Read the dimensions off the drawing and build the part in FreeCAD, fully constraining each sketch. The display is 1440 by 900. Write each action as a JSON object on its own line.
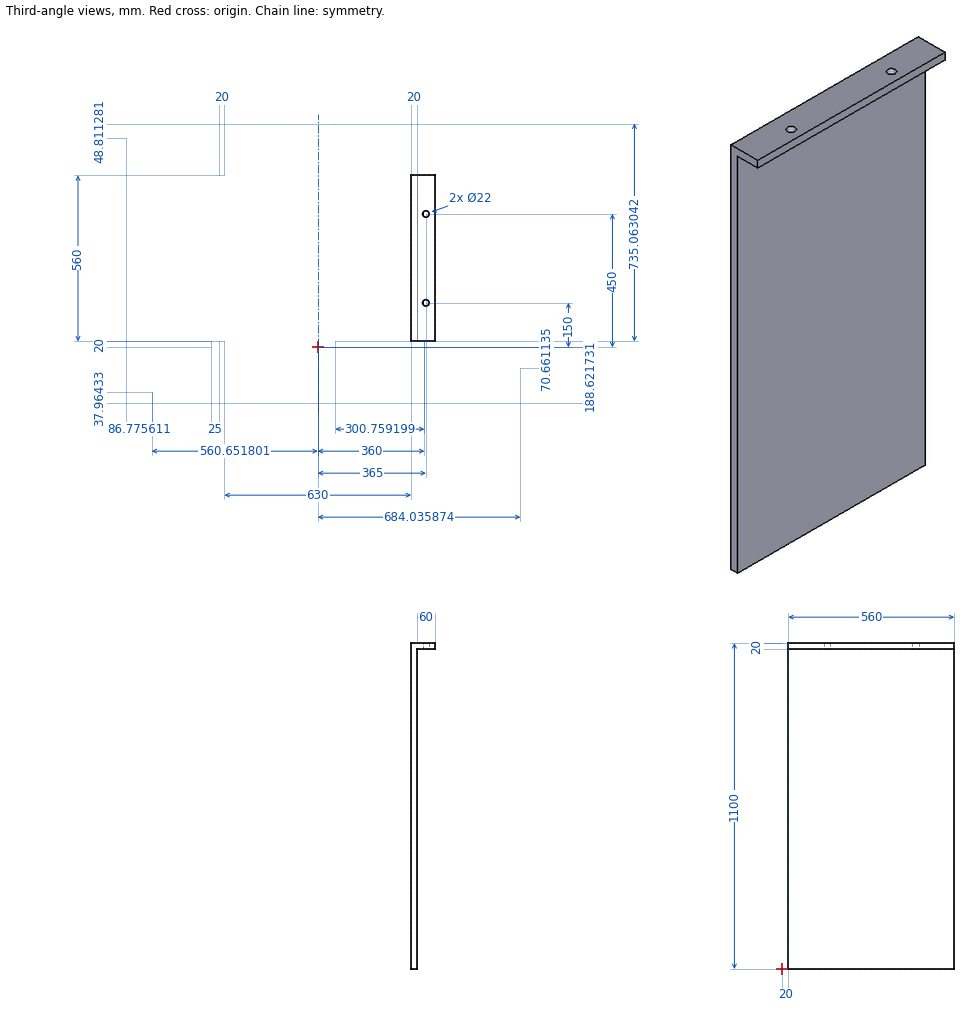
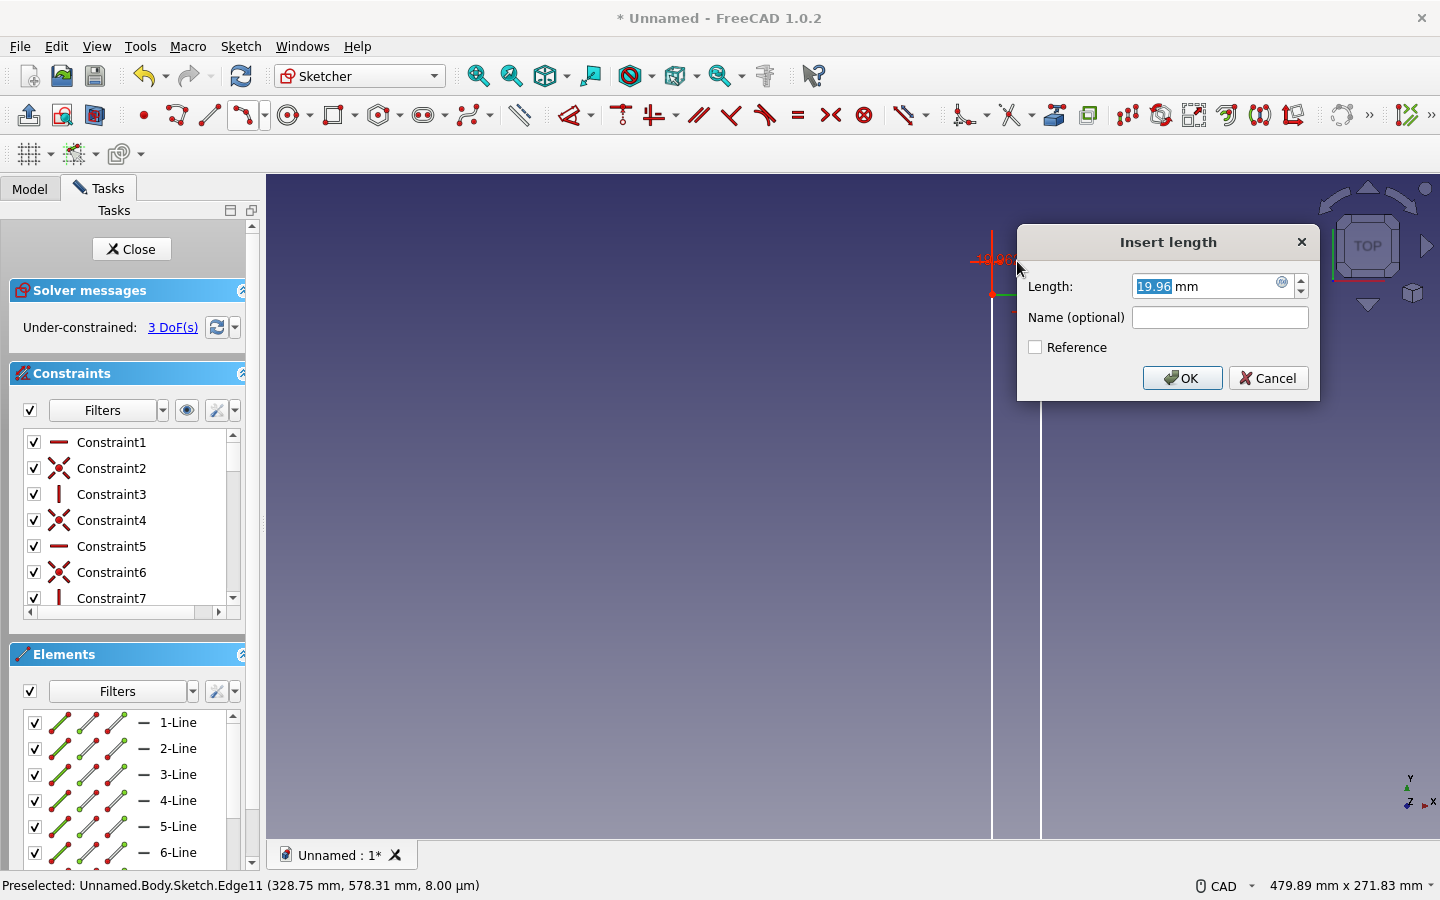
{"action": "type", "text": "20"}
{"action": "key", "text": "Return"}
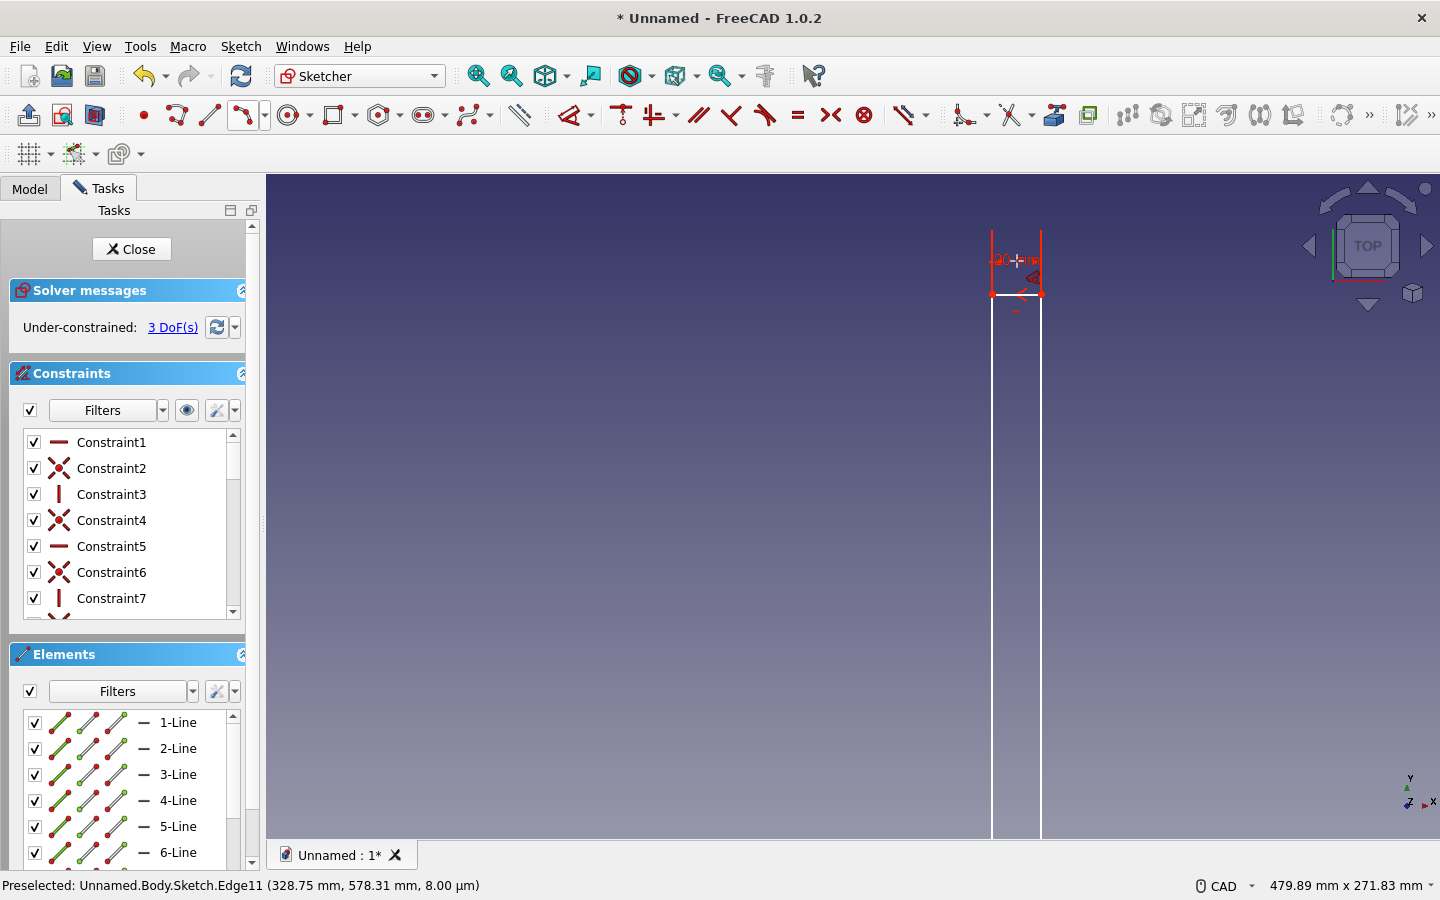
{"action": "scroll", "coordinate": [1027, 294], "scroll_direction": "down", "scroll_amount": 6}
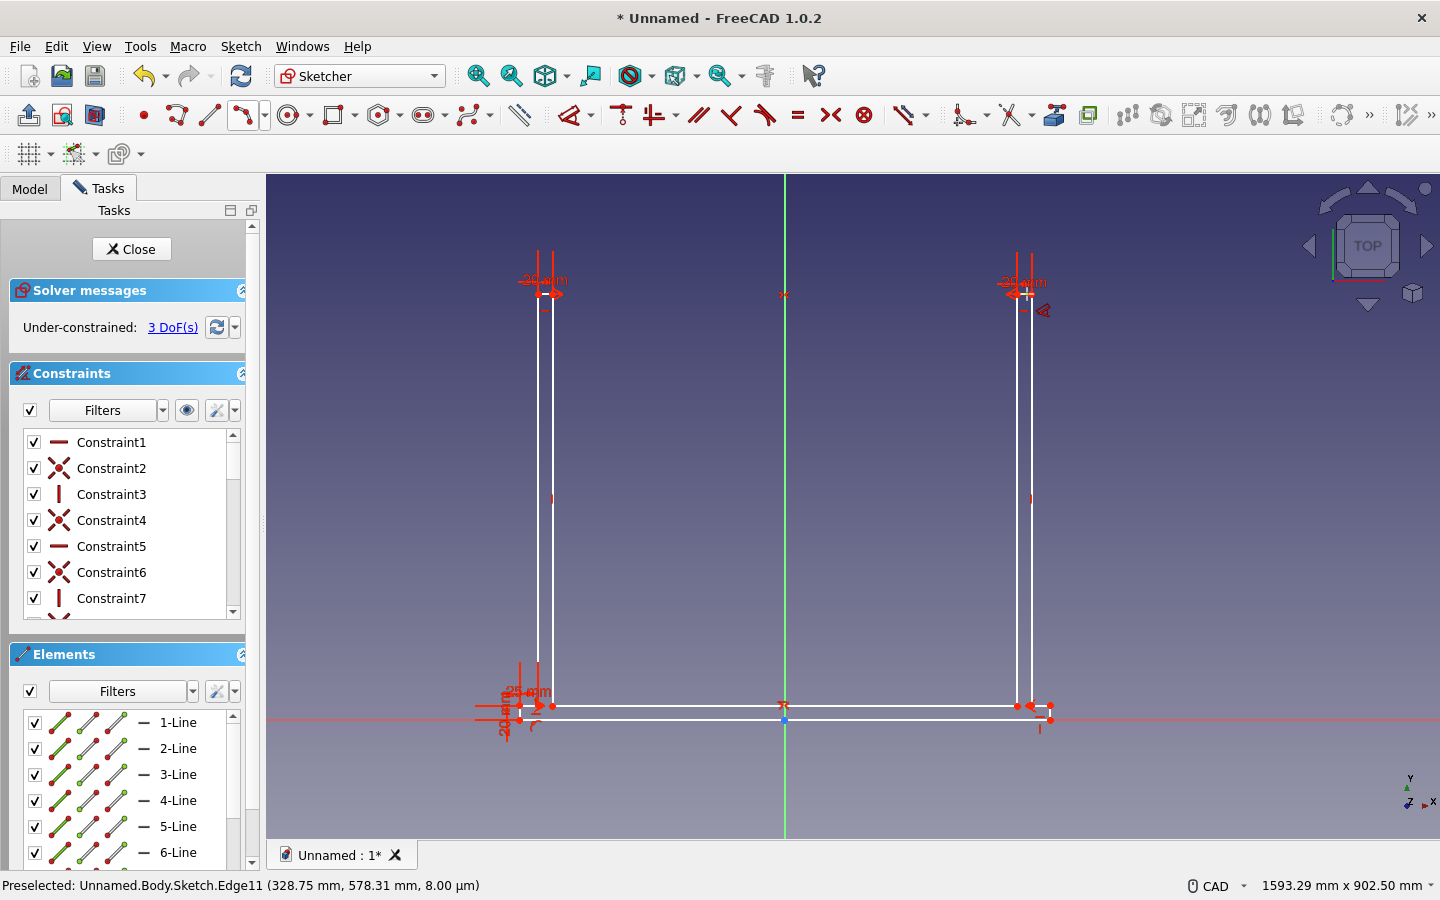
{"action": "left_click", "coordinate": [878, 706]}
{"action": "left_click", "coordinate": [678, 740]}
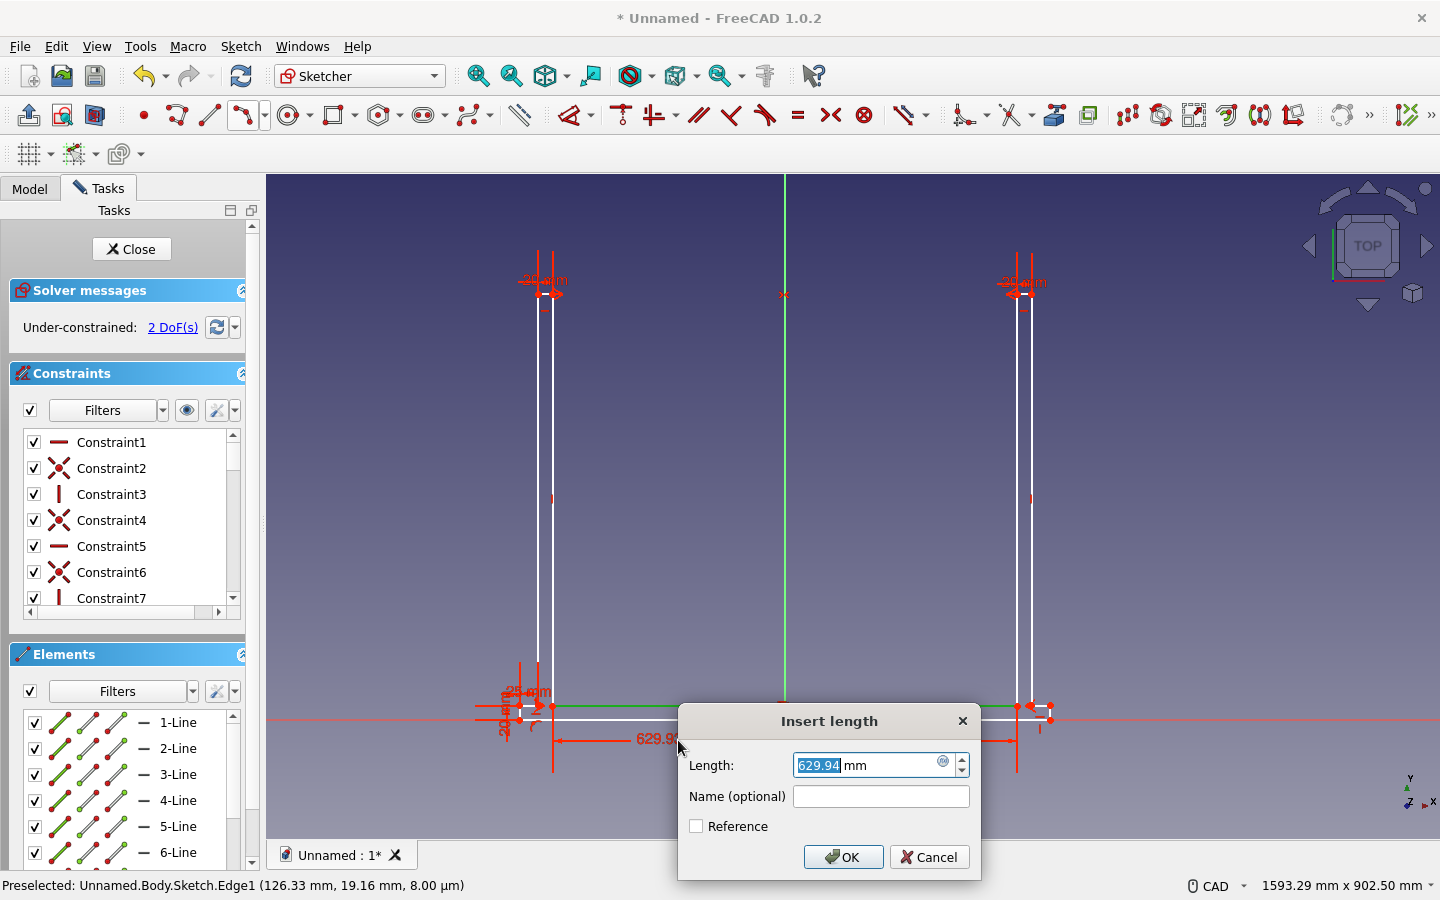
{"action": "type", "text": "630"}
{"action": "key", "text": "Return"}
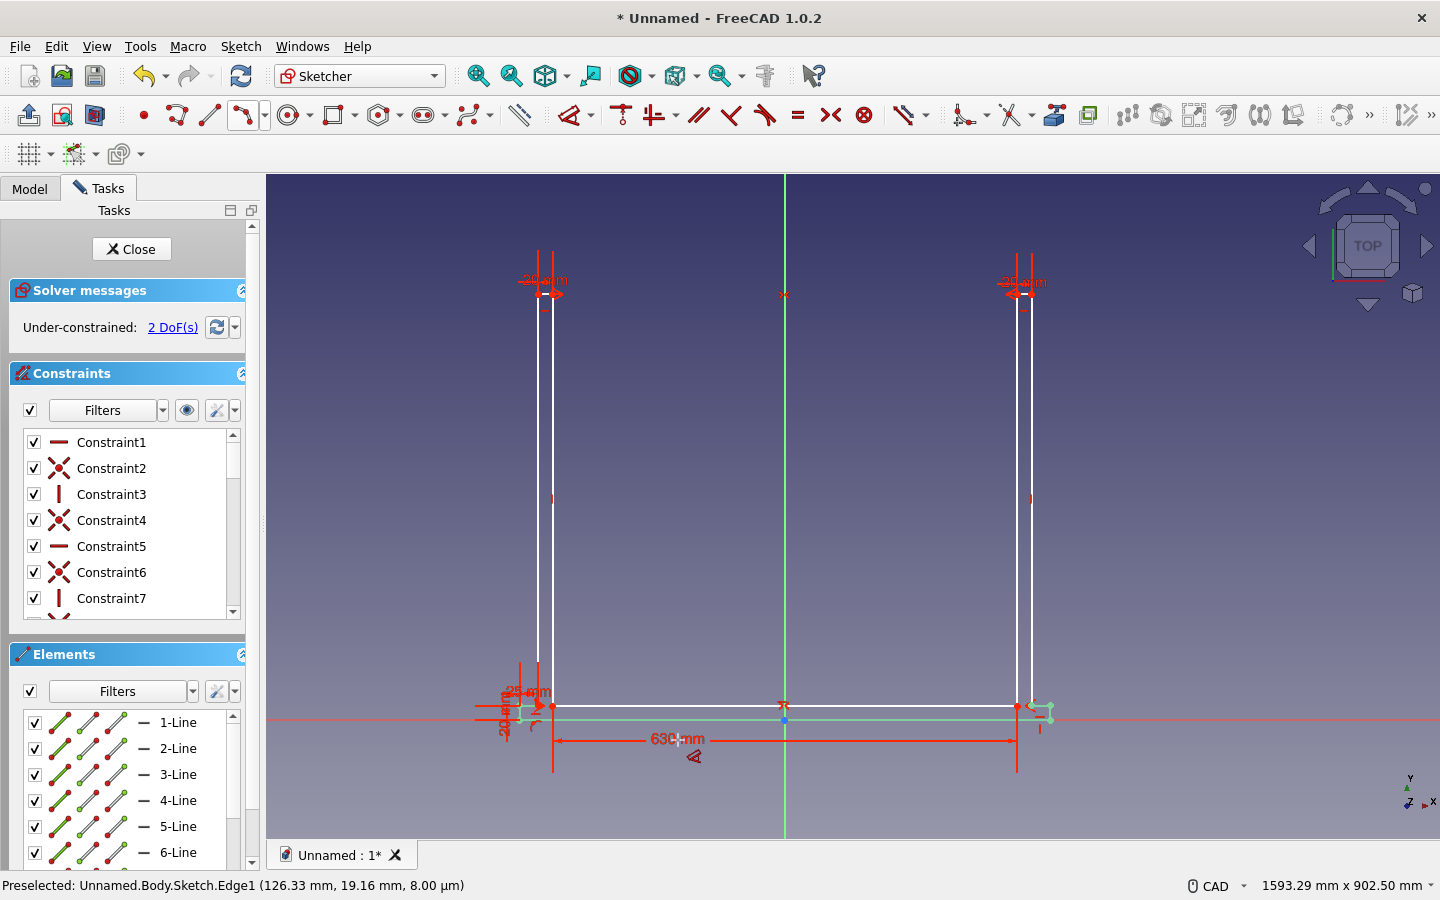
{"action": "left_click", "coordinate": [553, 583]}
{"action": "left_click", "coordinate": [519, 500]}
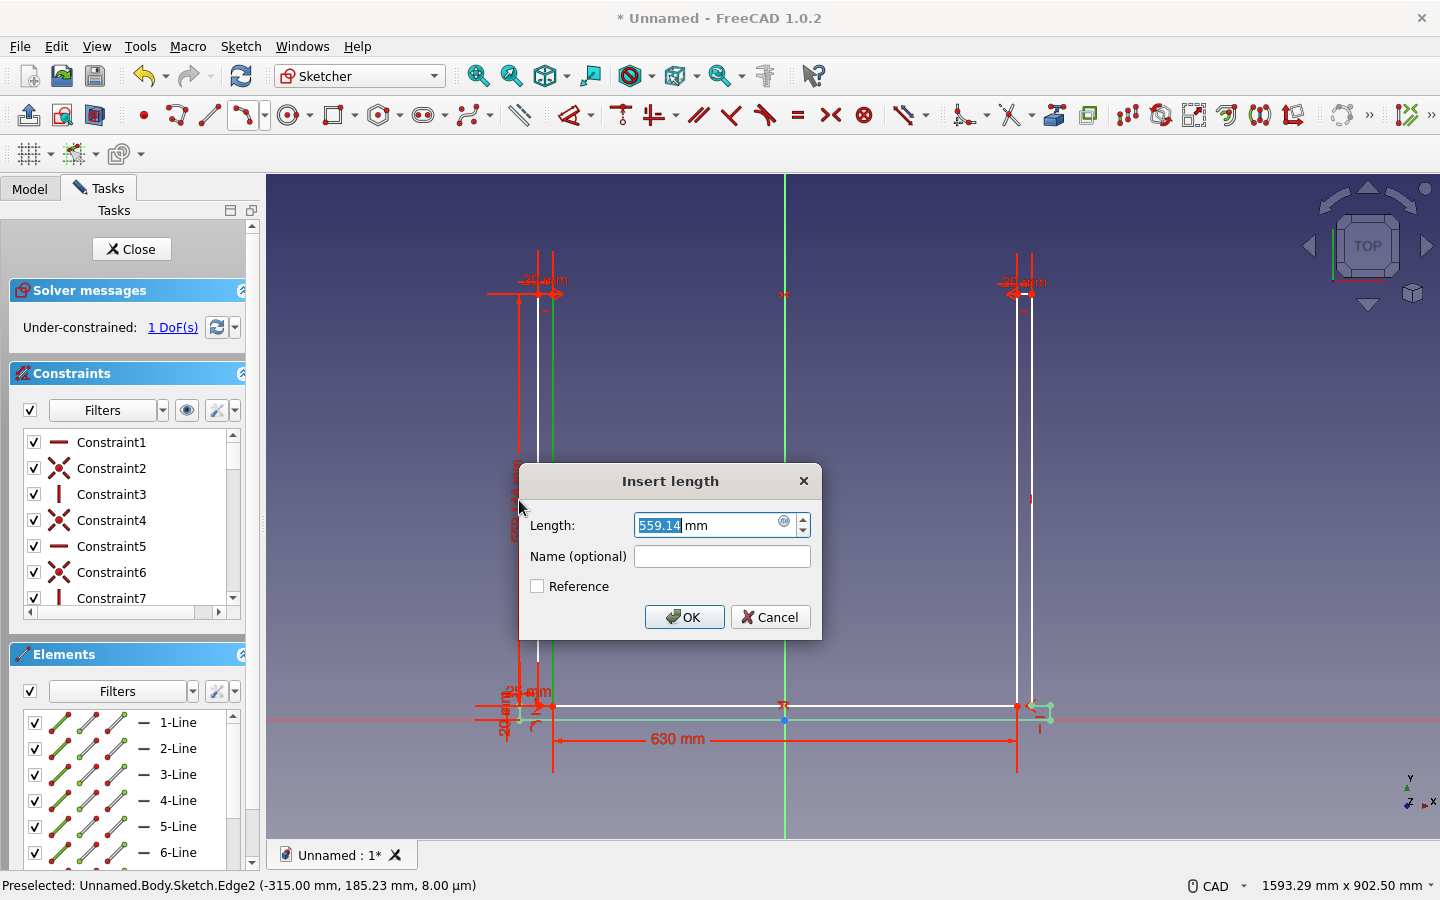
{"action": "type", "text": "560"}
{"action": "key", "text": "Return"}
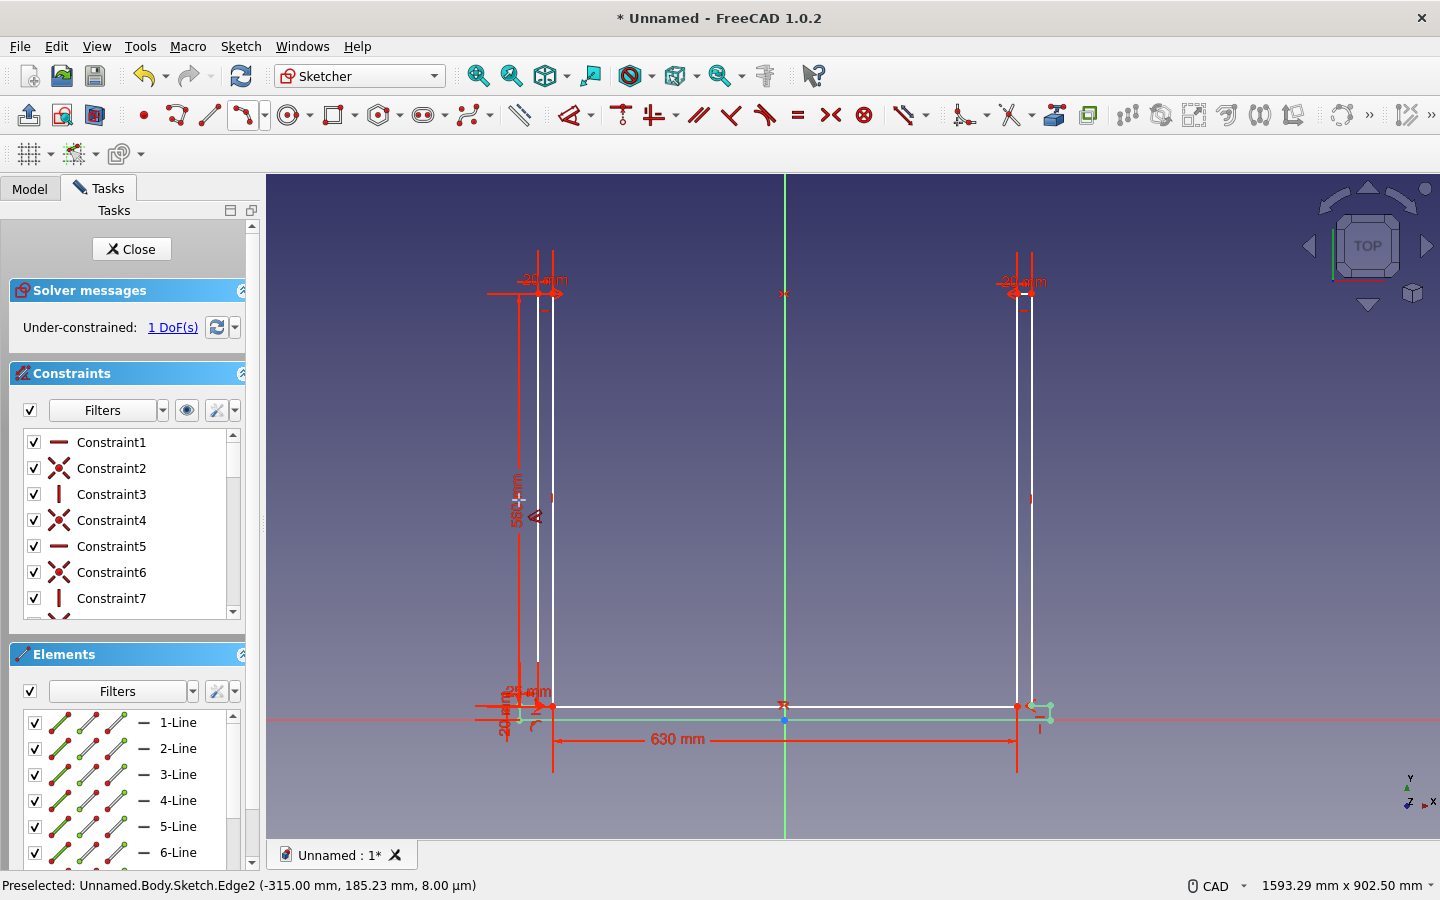
{"action": "left_click", "coordinate": [538, 417]}
{"action": "left_click", "coordinate": [504, 405]}